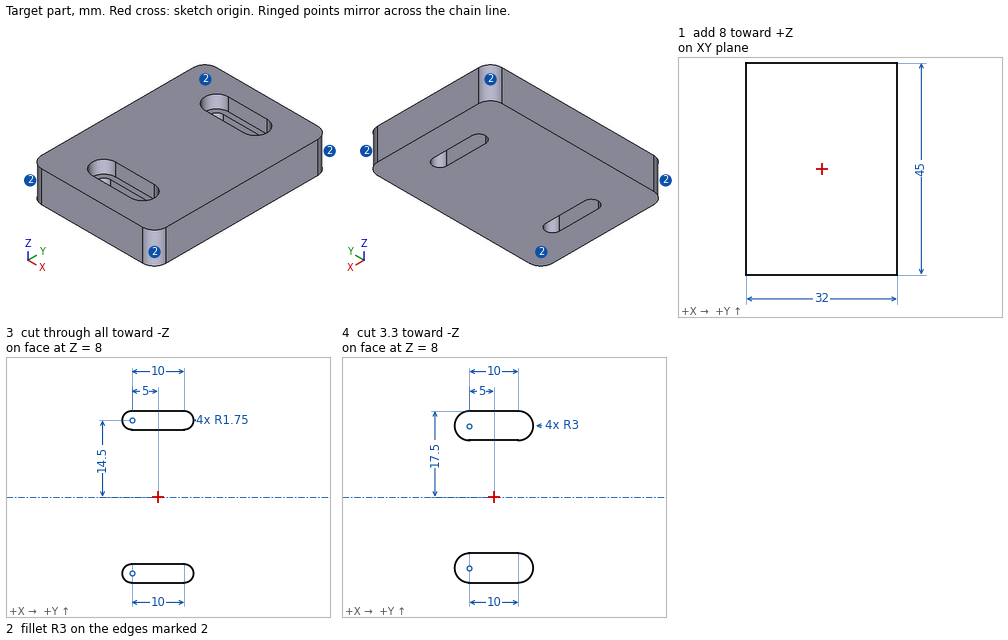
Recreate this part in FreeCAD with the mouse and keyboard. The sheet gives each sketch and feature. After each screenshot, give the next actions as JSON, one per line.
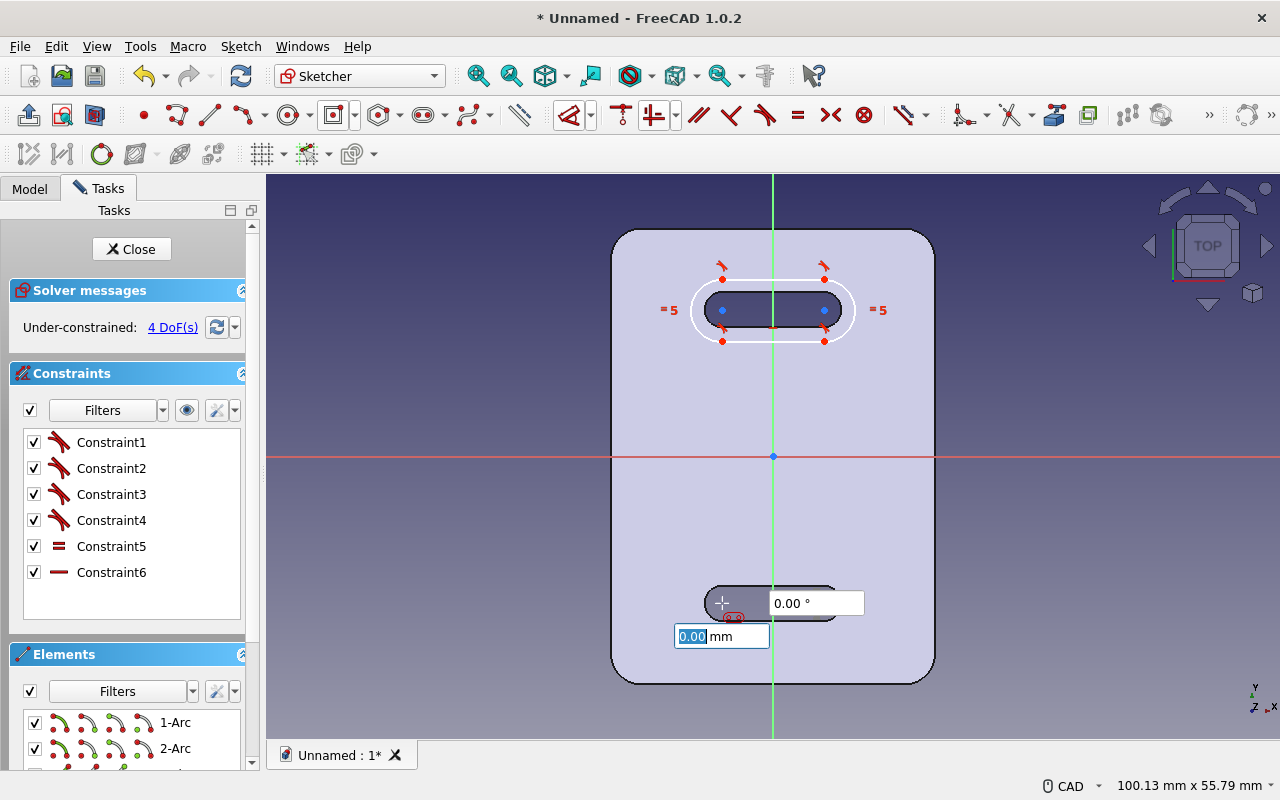
{"action": "left_click", "coordinate": [824, 603]}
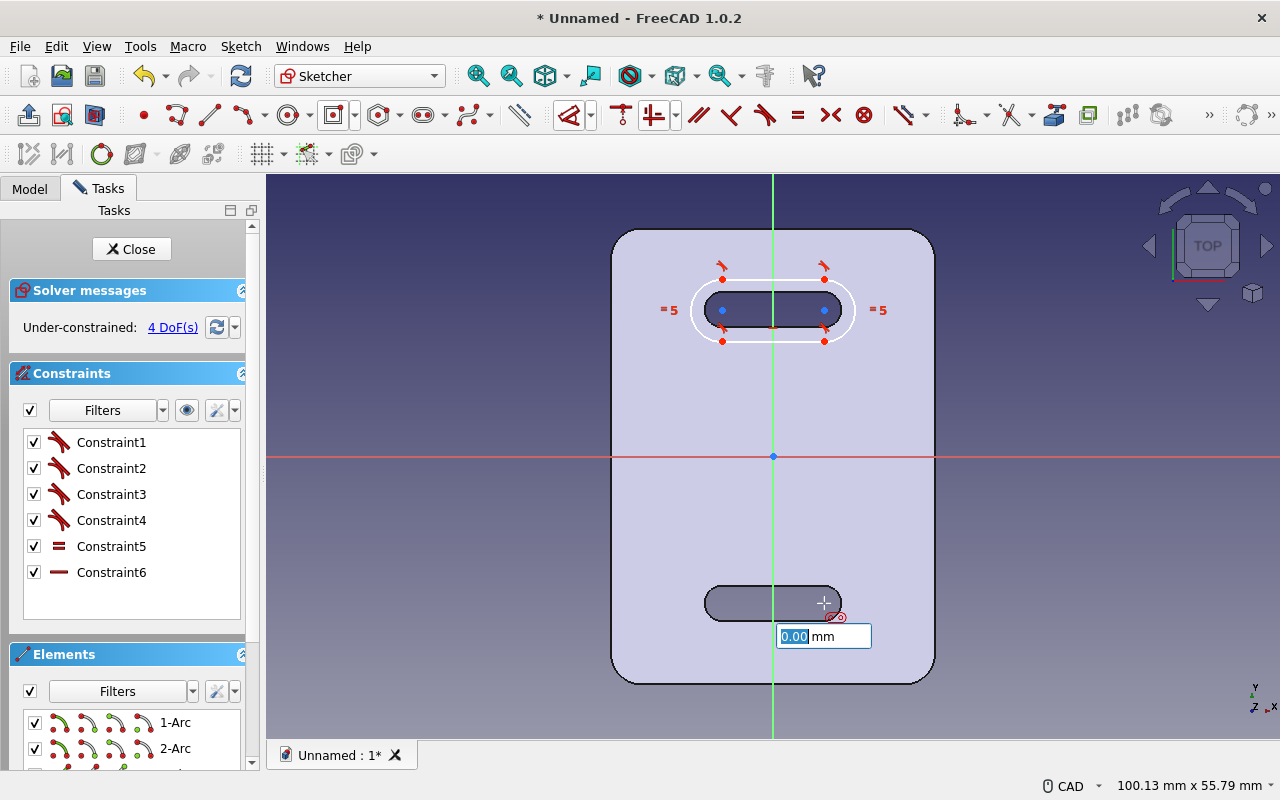
{"action": "left_click", "coordinate": [788, 573]}
{"action": "key", "text": "Escape"}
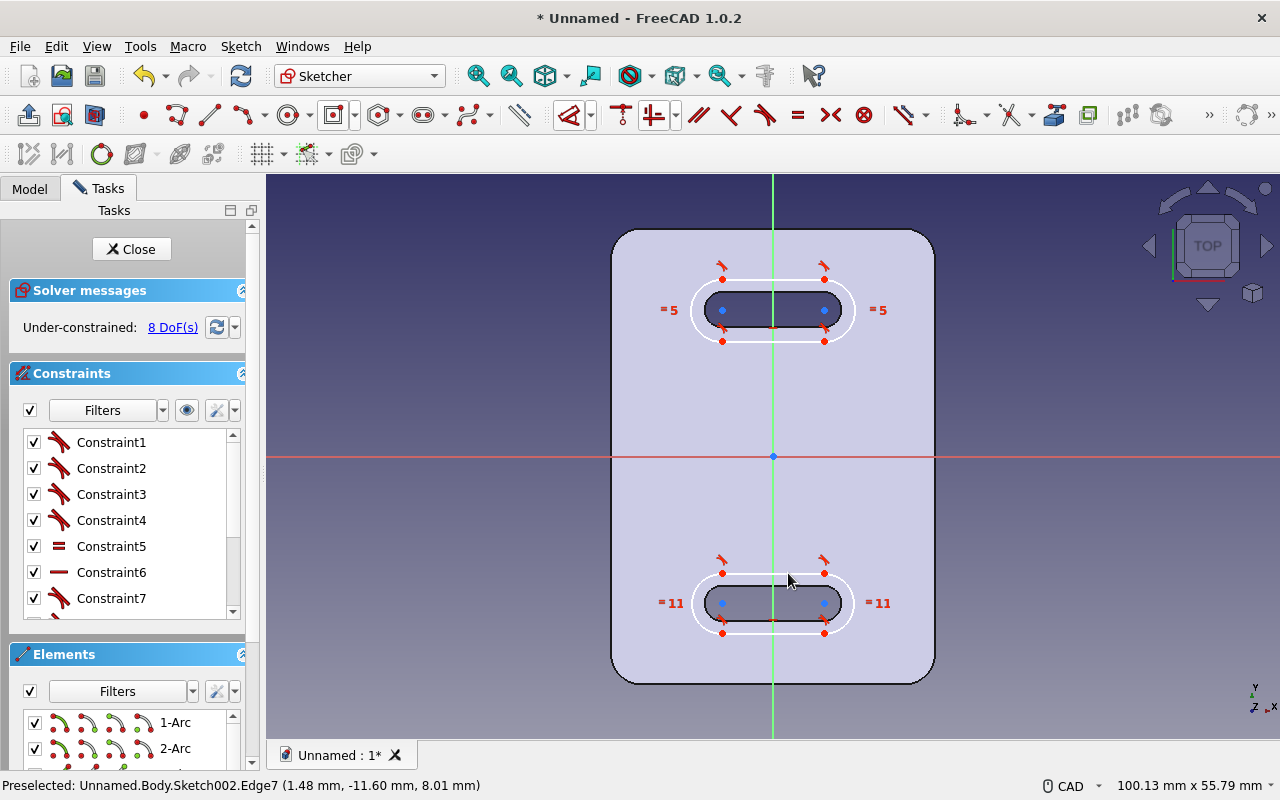
{"action": "left_click", "coordinate": [697, 293]}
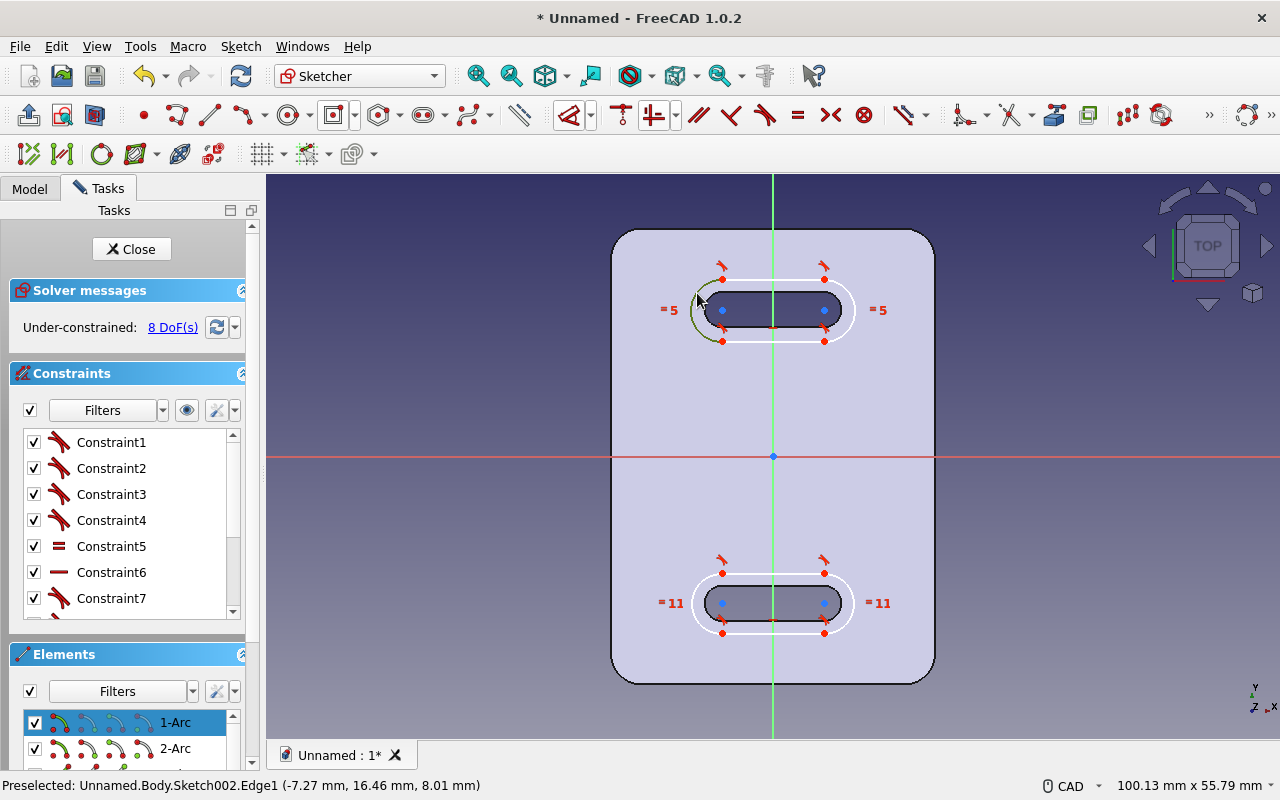
{"action": "left_click", "coordinate": [698, 586]}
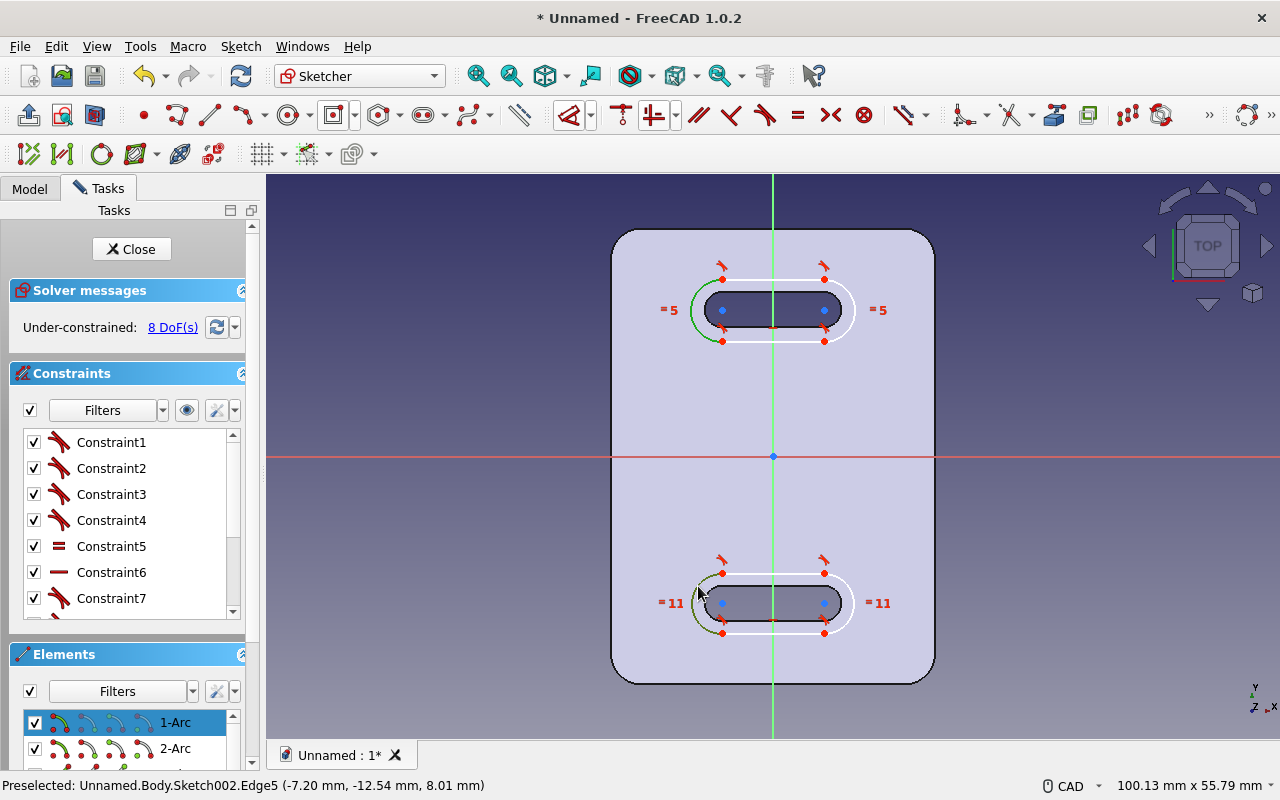
{"action": "left_click", "coordinate": [798, 116]}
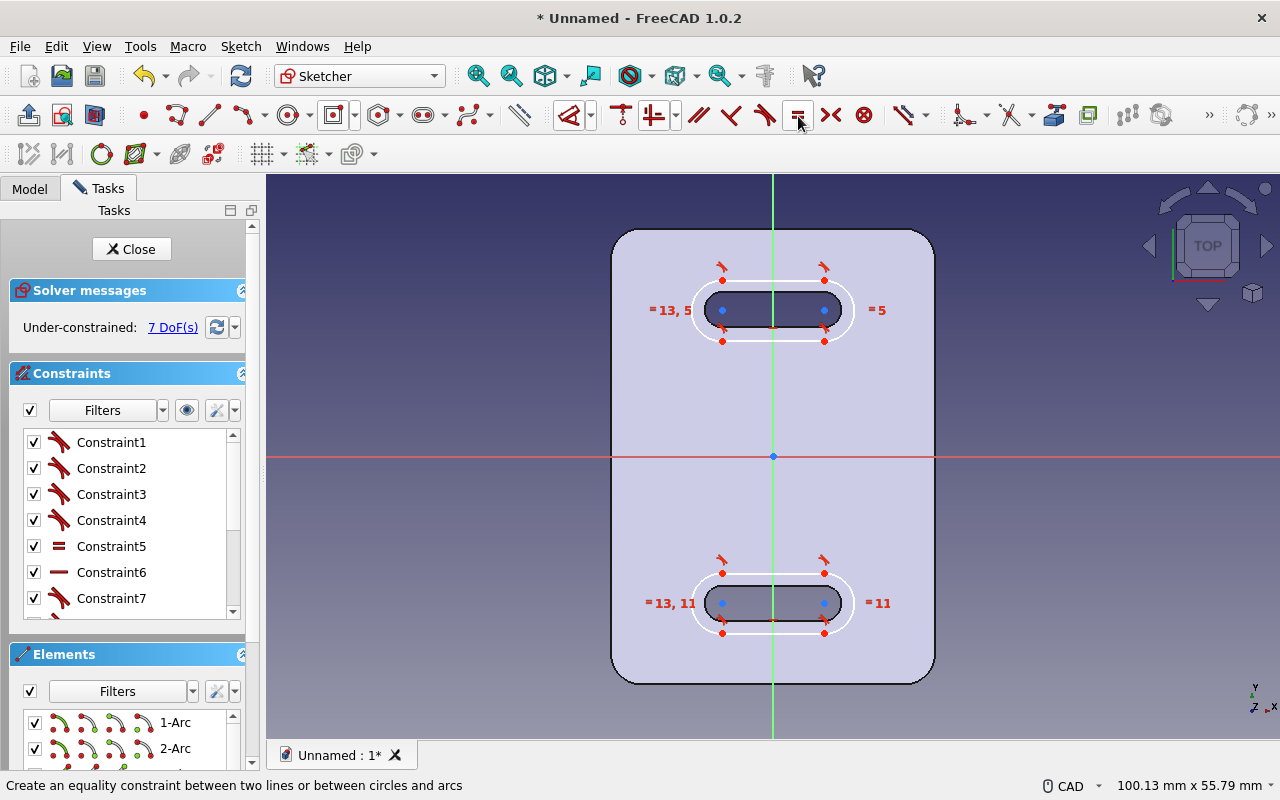
{"action": "left_click", "coordinate": [722, 311]}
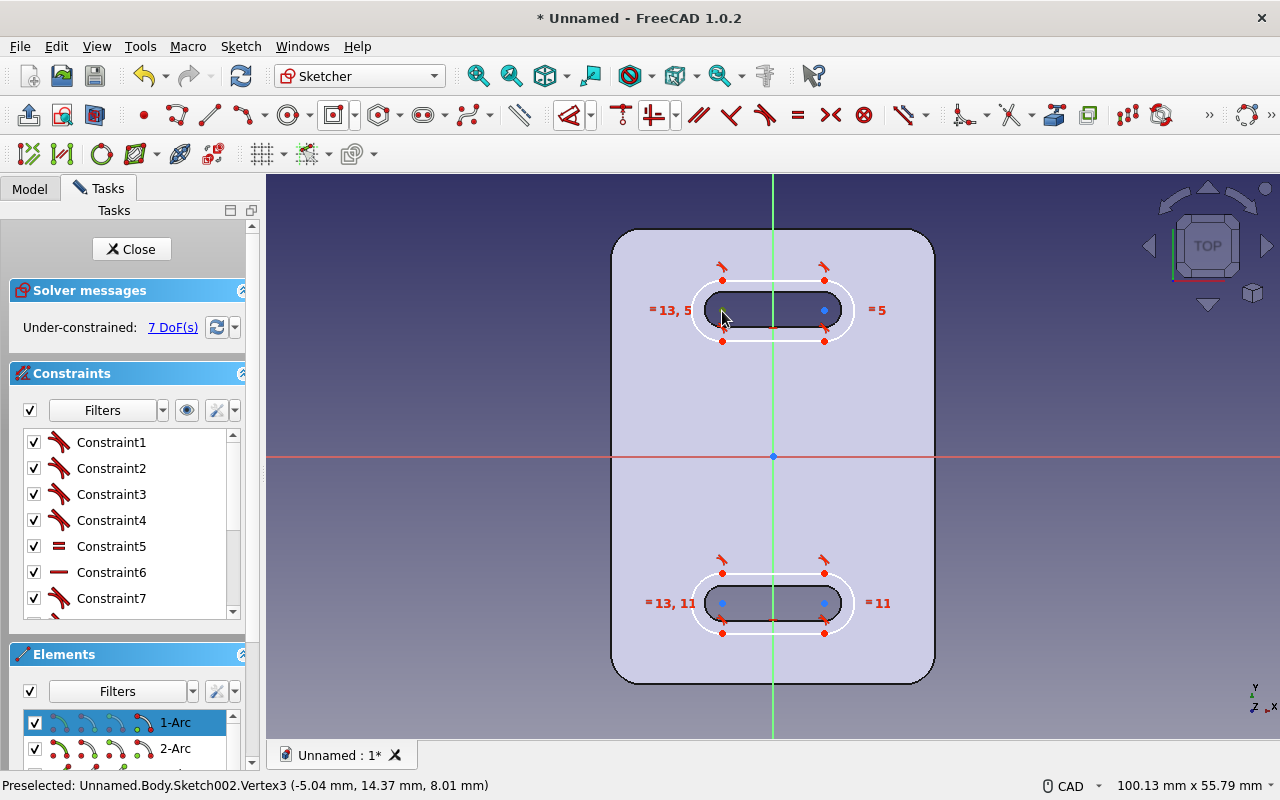
{"action": "left_click", "coordinate": [722, 604]}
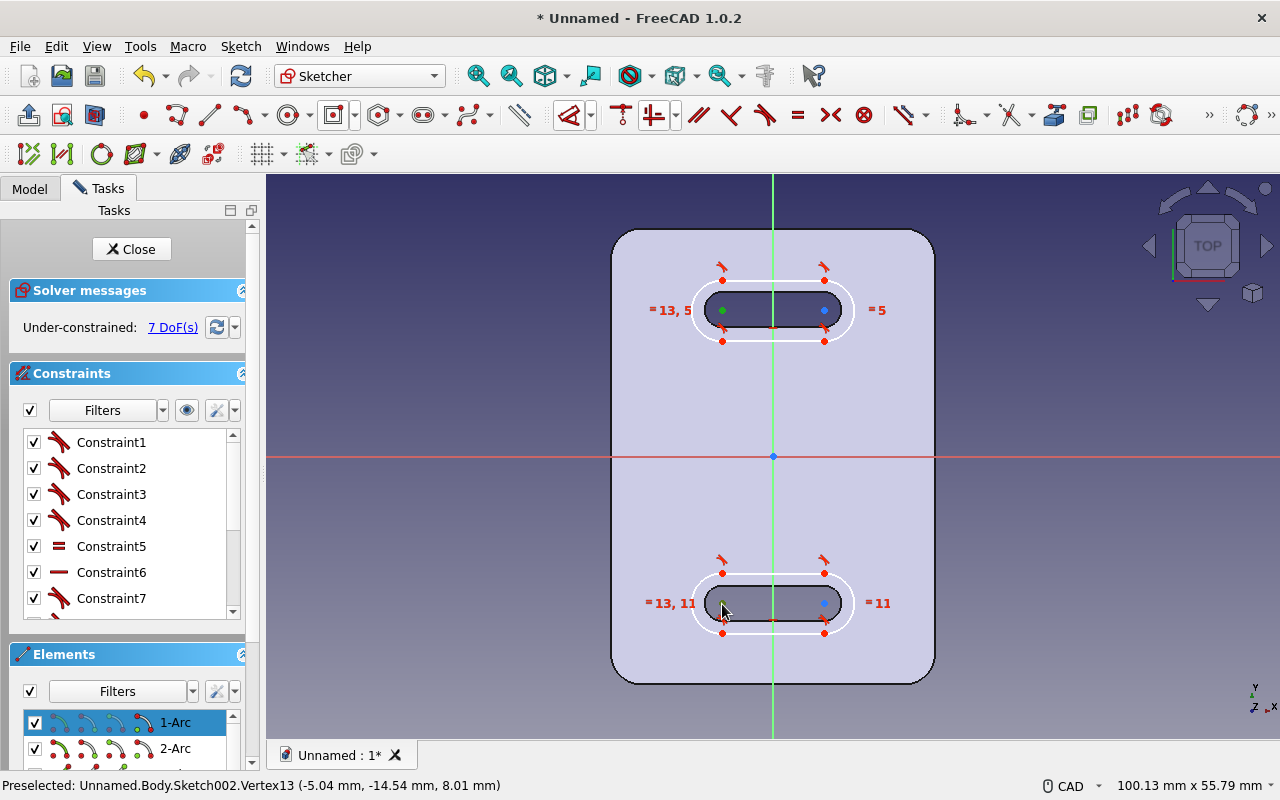
{"action": "left_click", "coordinate": [353, 456]}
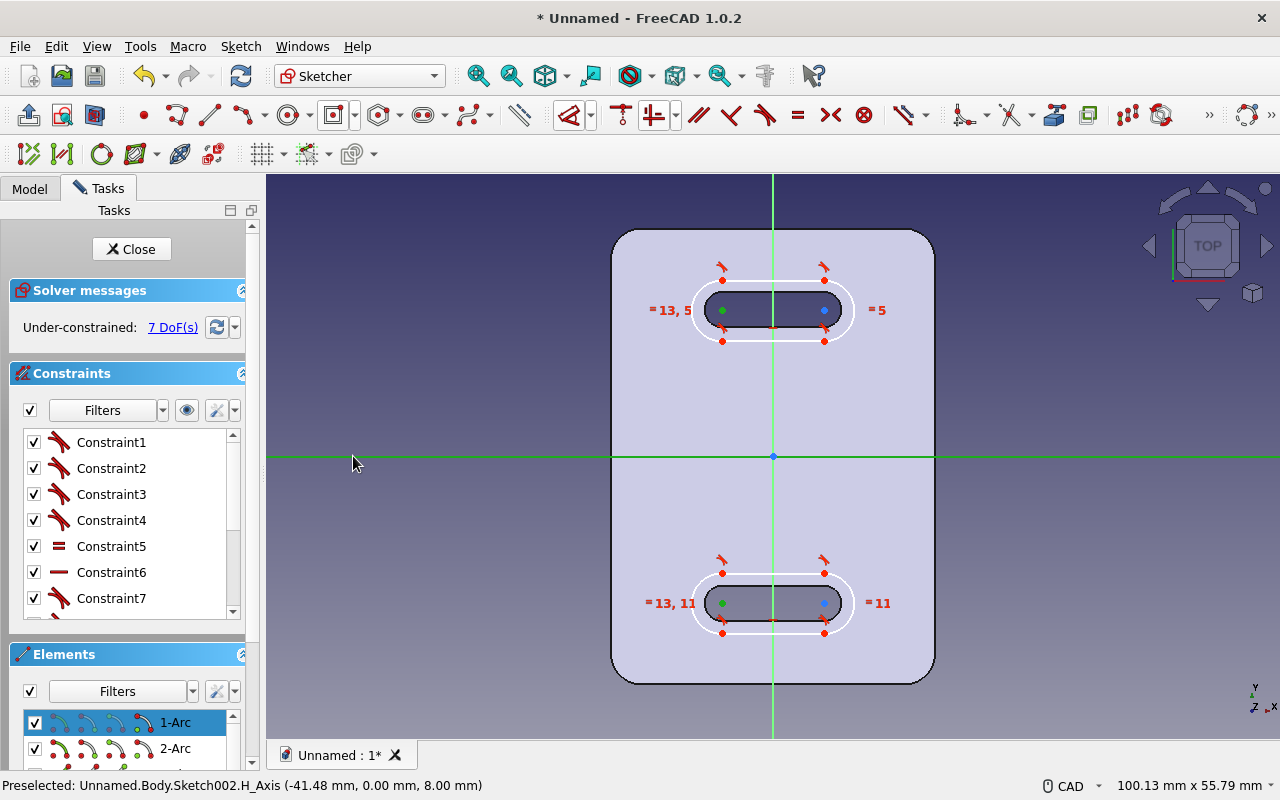
{"action": "left_click", "coordinate": [831, 116]}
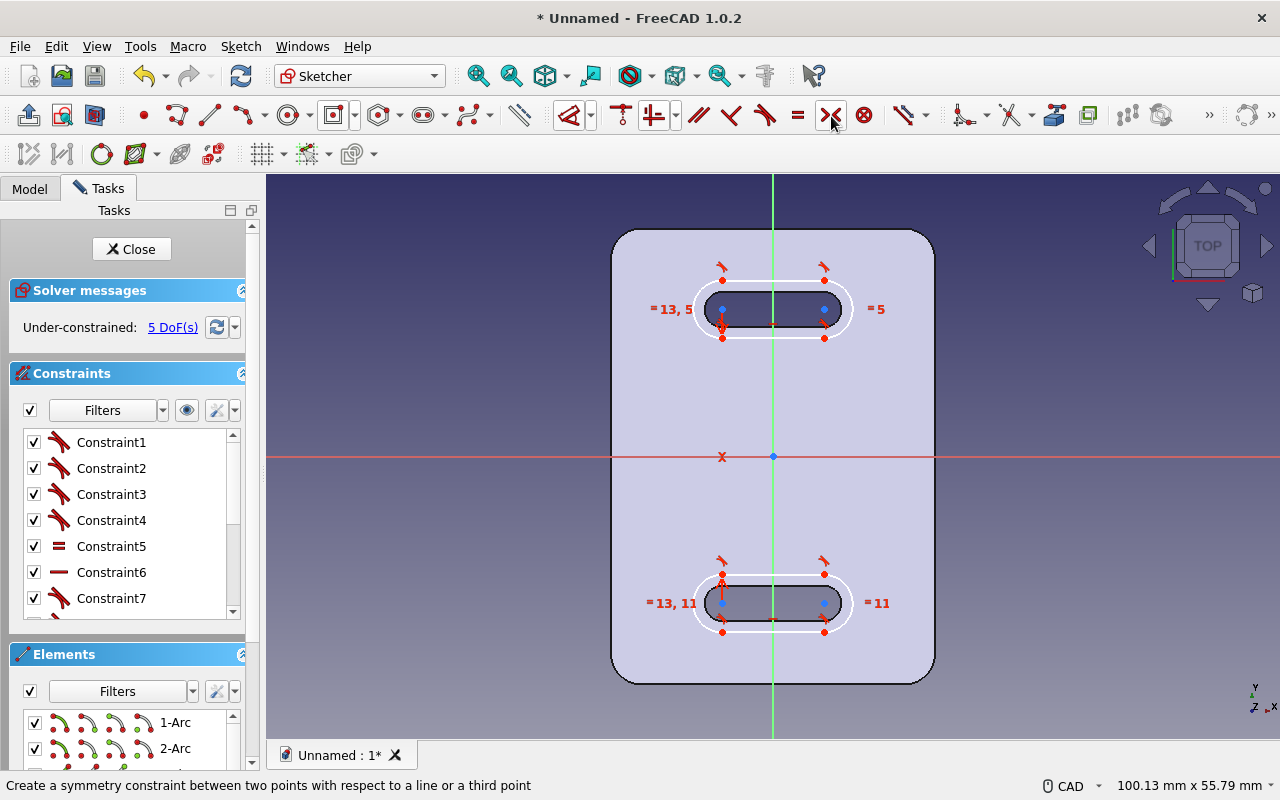
{"action": "scroll", "coordinate": [699, 293], "scroll_direction": "up", "scroll_amount": 2}